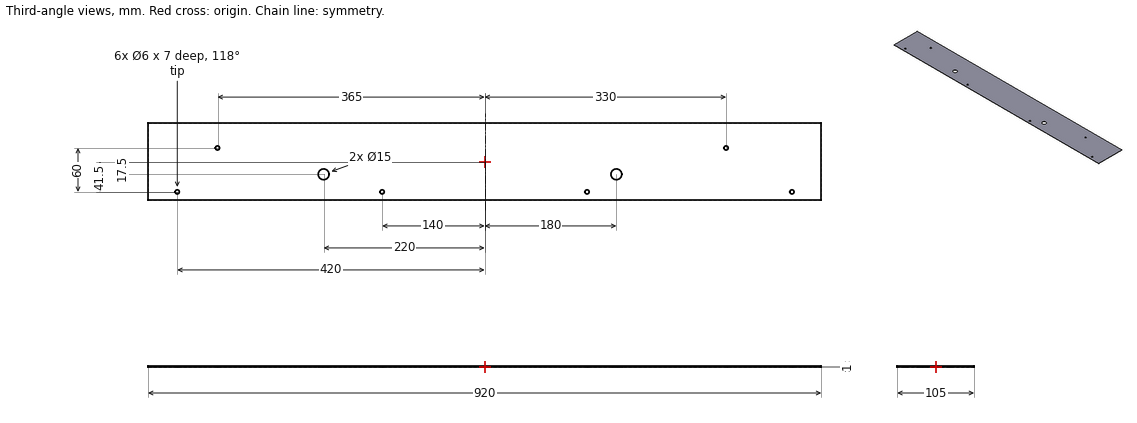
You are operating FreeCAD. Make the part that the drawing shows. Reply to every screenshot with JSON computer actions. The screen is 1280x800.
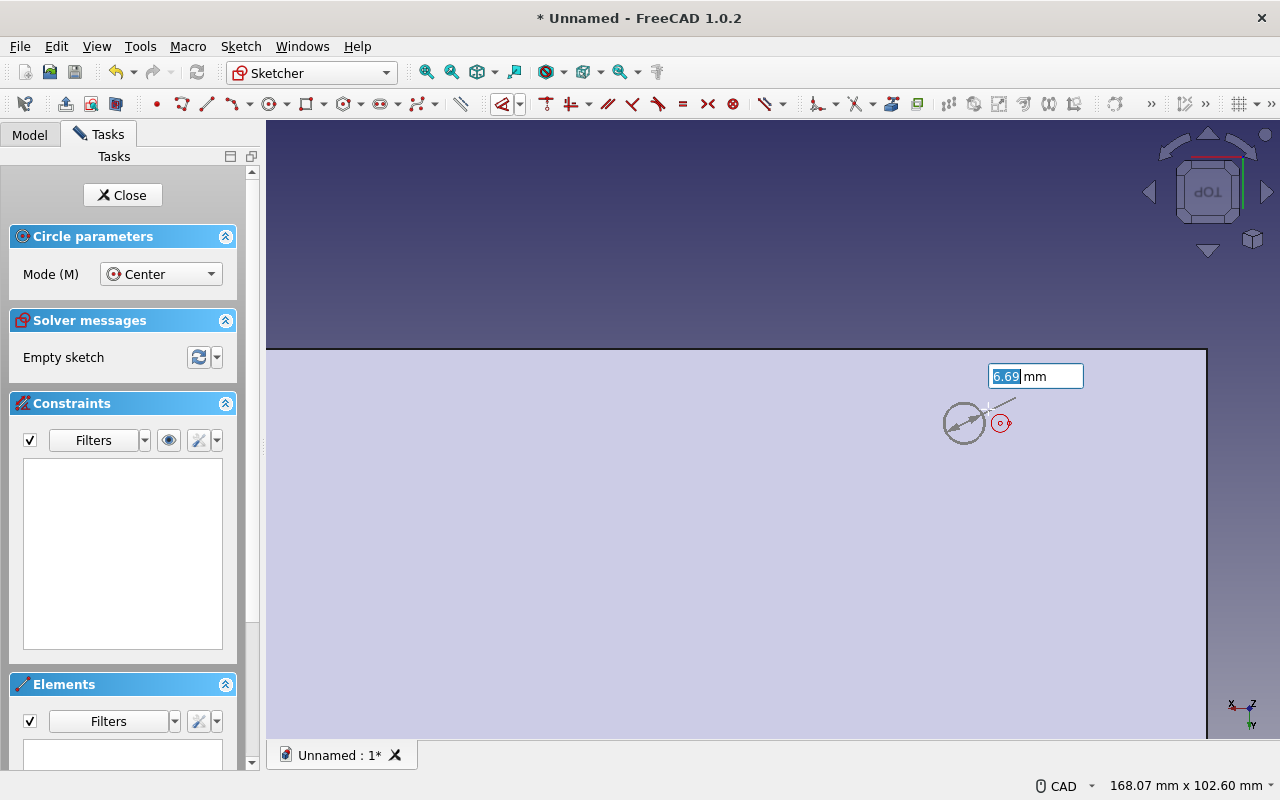
{"action": "left_click", "coordinate": [978, 402]}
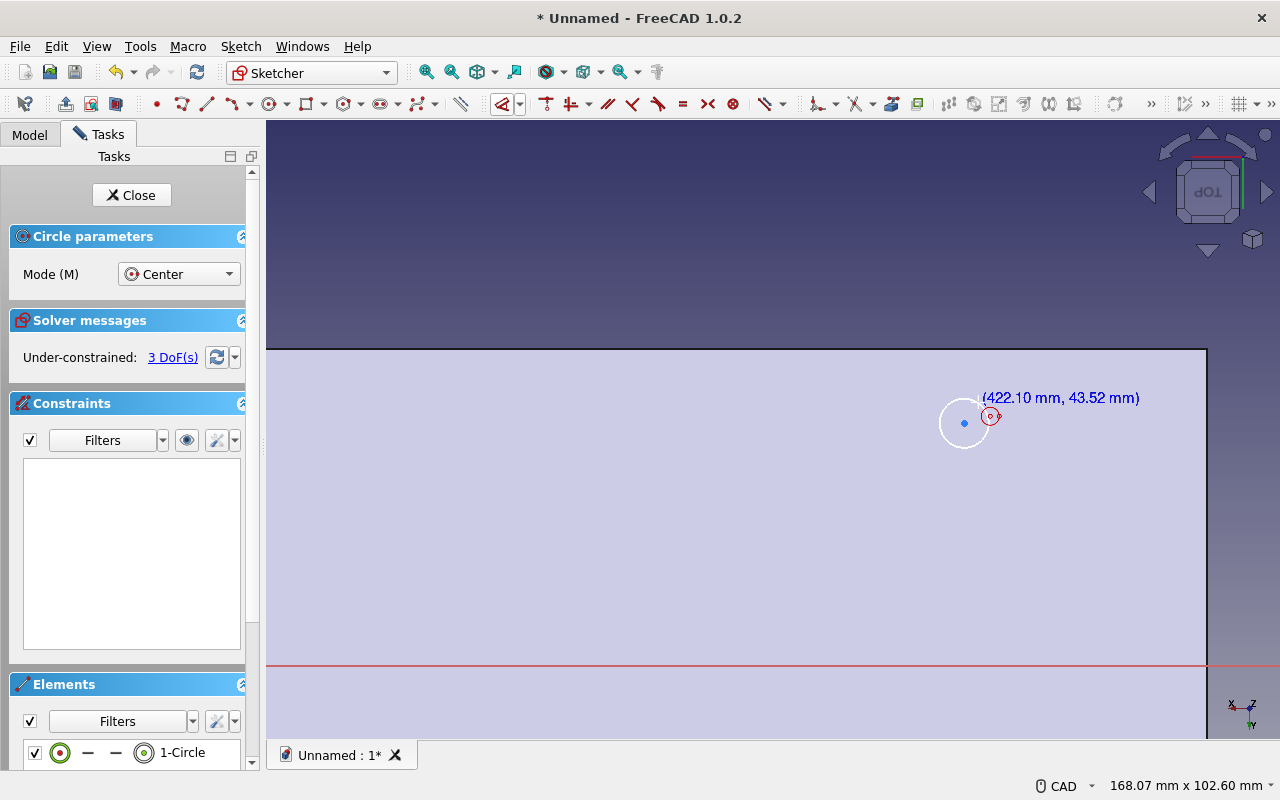
{"action": "scroll", "coordinate": [988, 409], "scroll_direction": "down", "scroll_amount": 11}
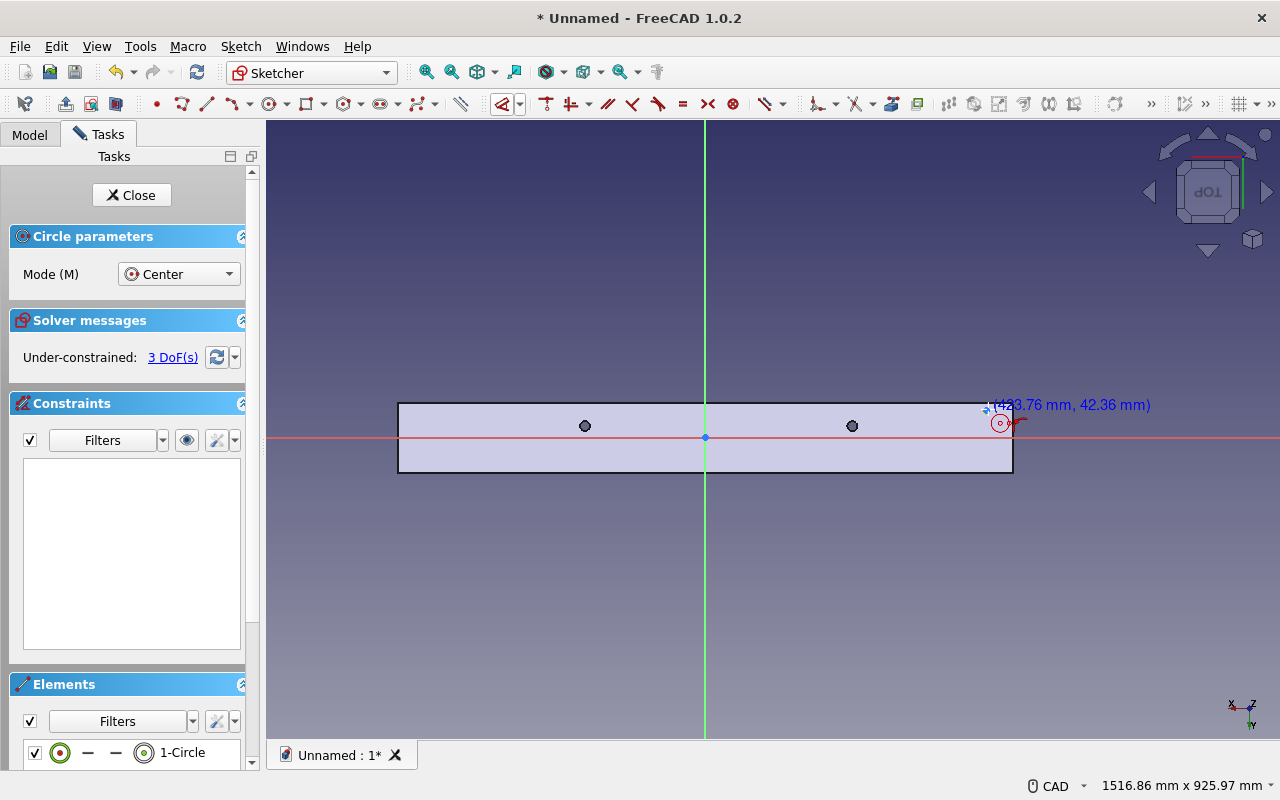
{"action": "scroll", "coordinate": [799, 410], "scroll_direction": "up", "scroll_amount": 13}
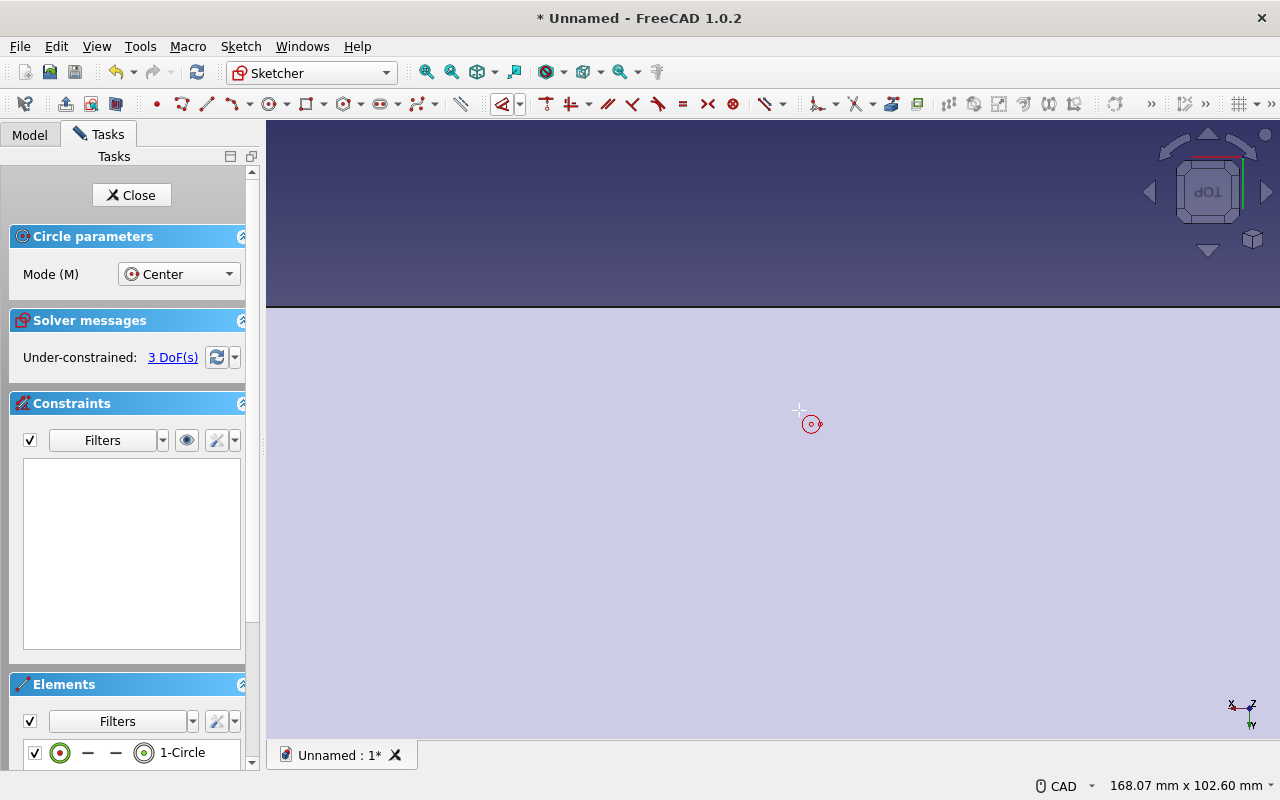
{"action": "scroll", "coordinate": [799, 410], "scroll_direction": "down", "scroll_amount": 13}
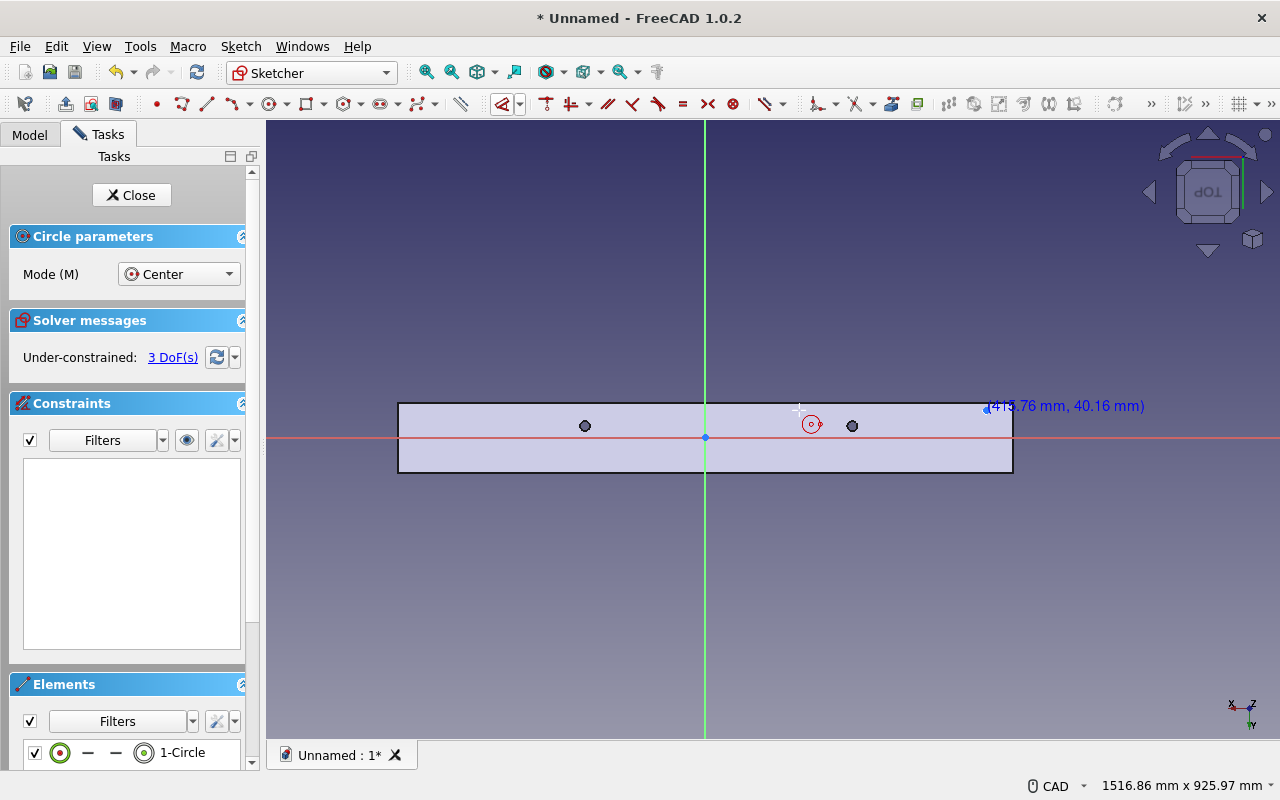
{"action": "left_click", "coordinate": [799, 410]}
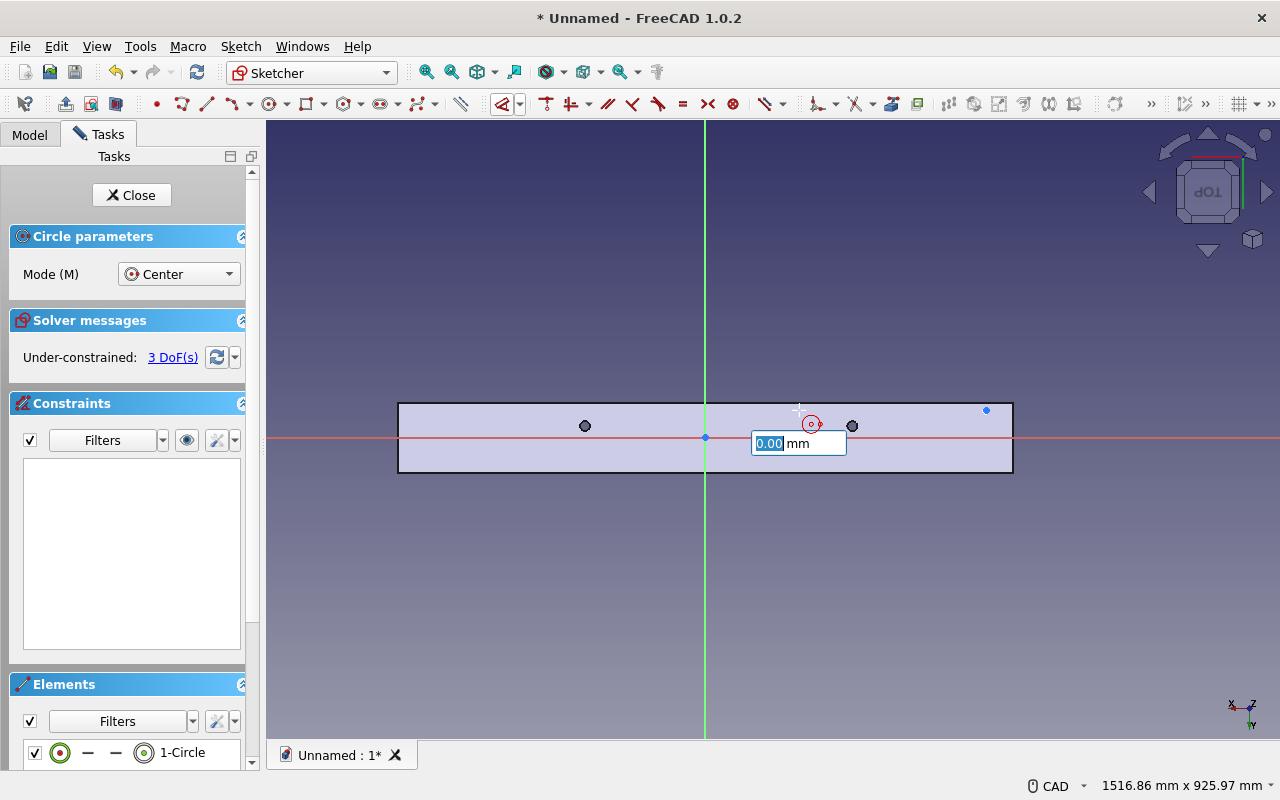
{"action": "scroll", "coordinate": [800, 409], "scroll_direction": "up", "scroll_amount": 11}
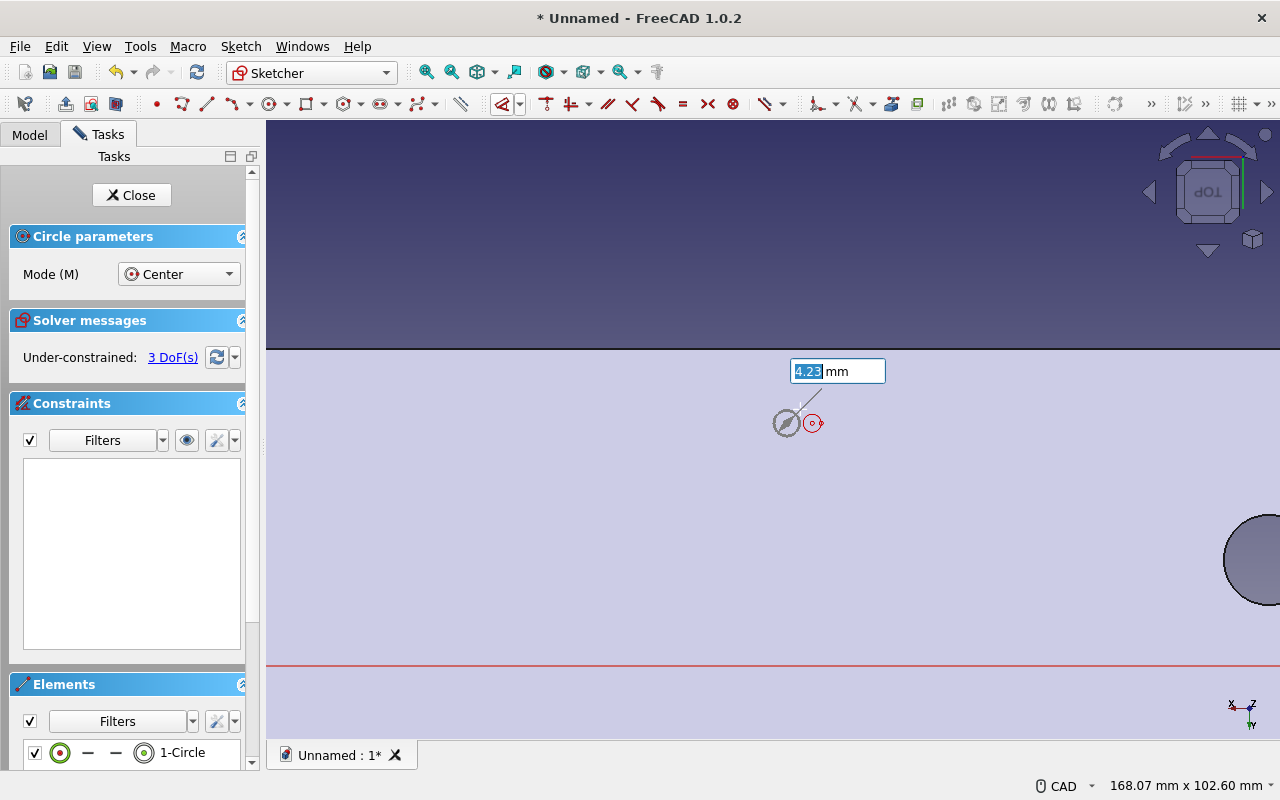
{"action": "left_click", "coordinate": [799, 402]}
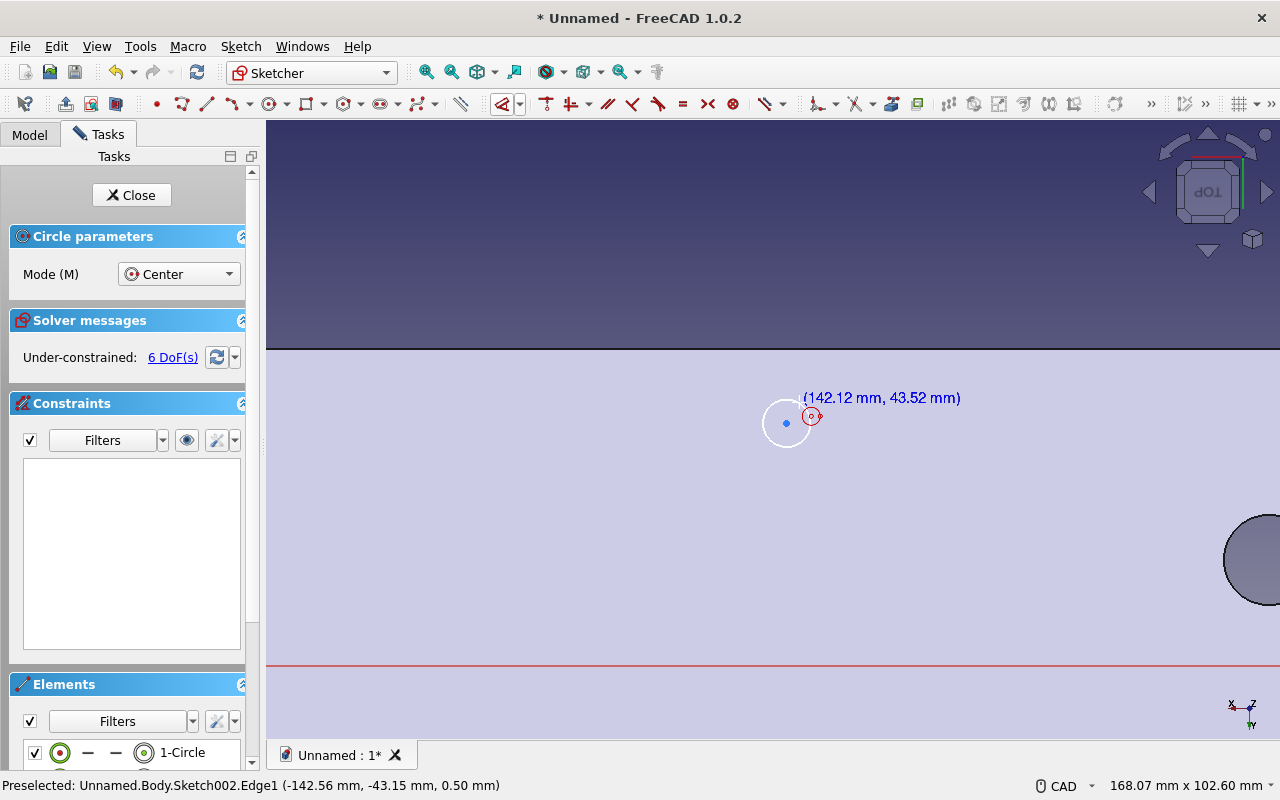
{"action": "scroll", "coordinate": [800, 409], "scroll_direction": "down", "scroll_amount": 11}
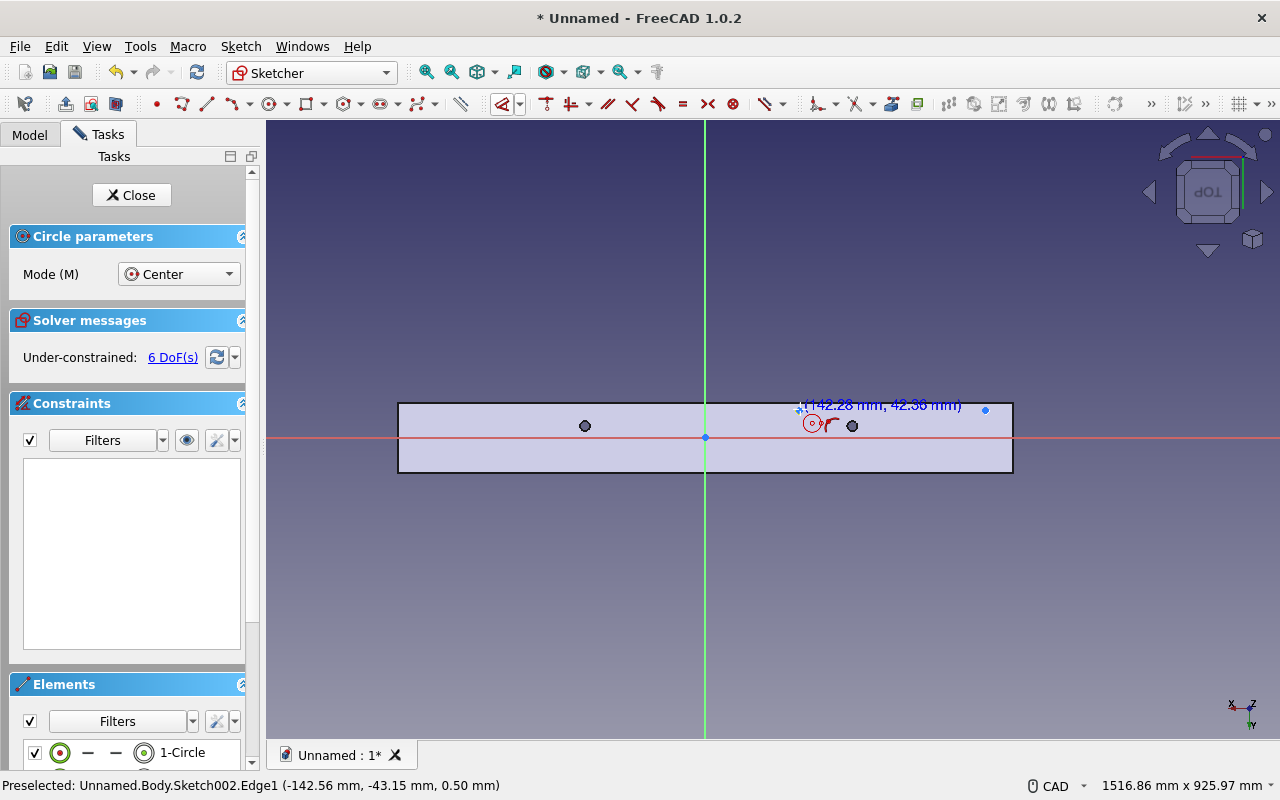
{"action": "scroll", "coordinate": [612, 410], "scroll_direction": "up", "scroll_amount": 13}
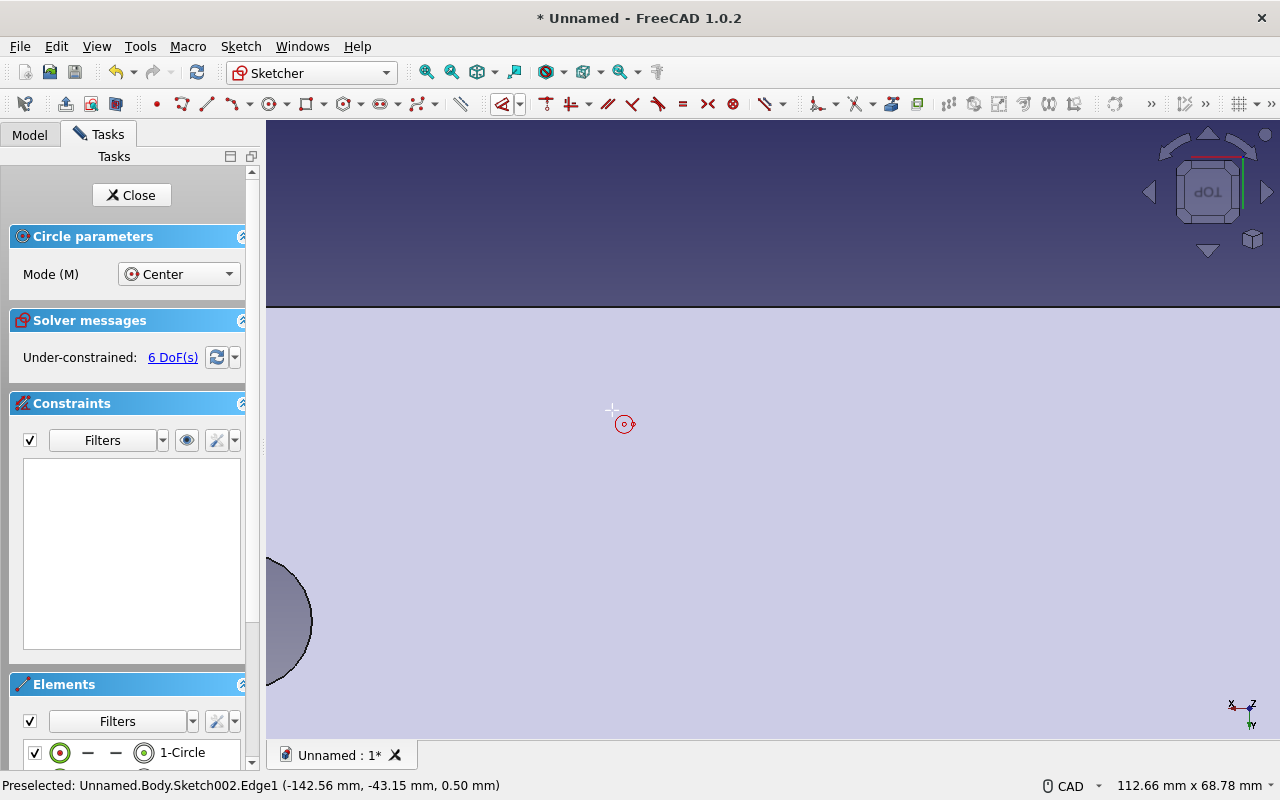
{"action": "scroll", "coordinate": [611, 410], "scroll_direction": "down", "scroll_amount": 13}